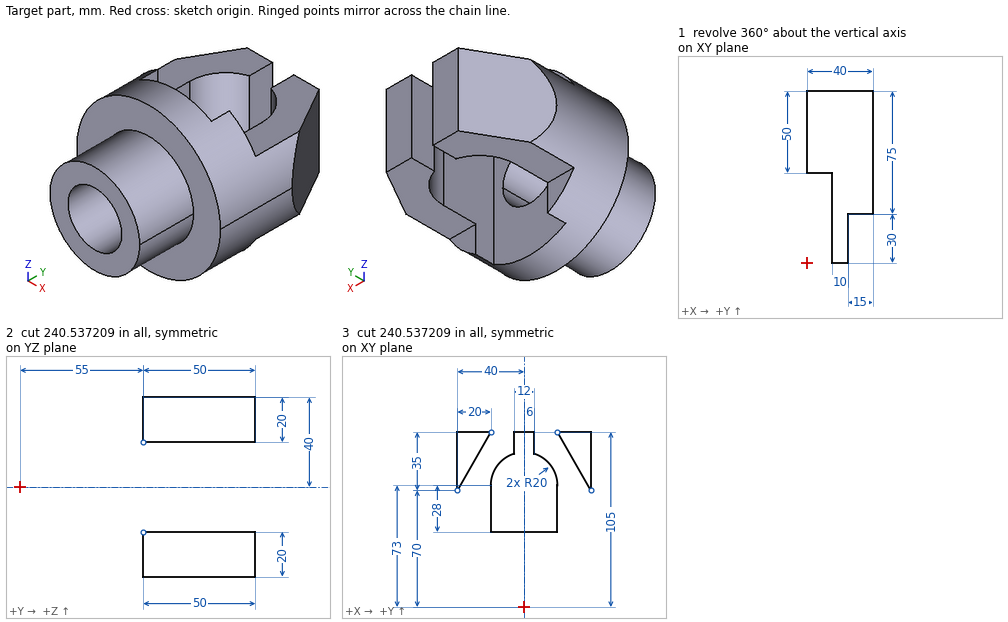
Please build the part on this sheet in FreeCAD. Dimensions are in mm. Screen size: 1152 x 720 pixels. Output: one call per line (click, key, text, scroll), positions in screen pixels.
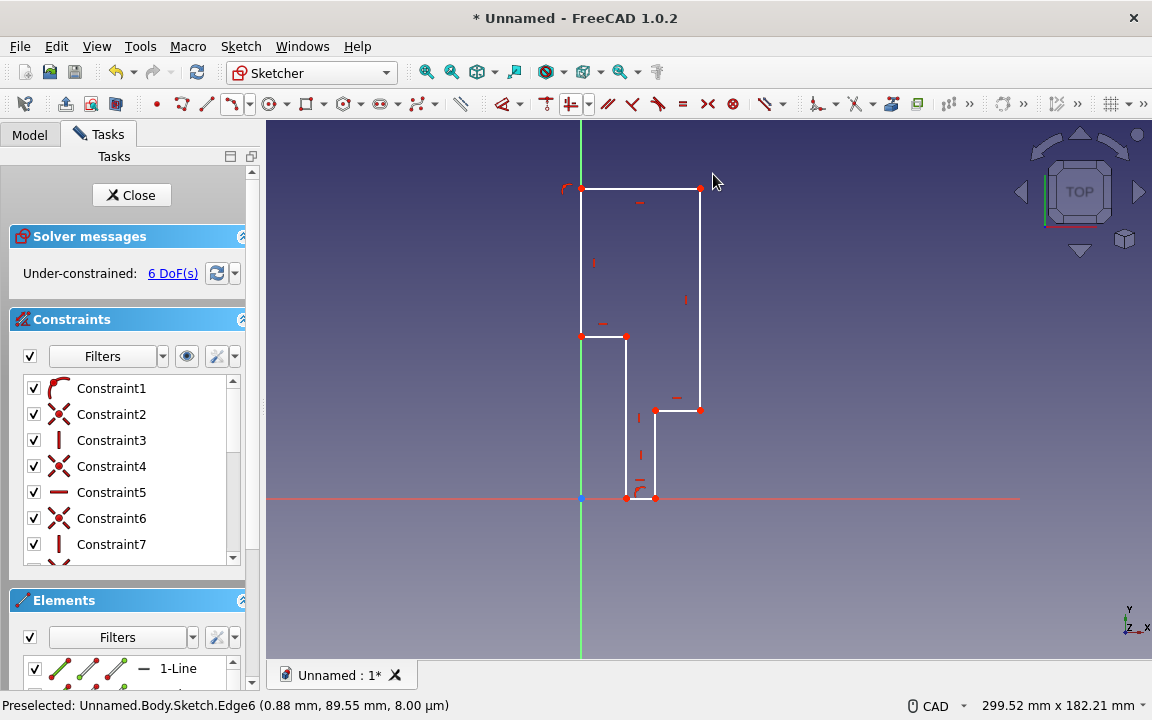
click(502, 104)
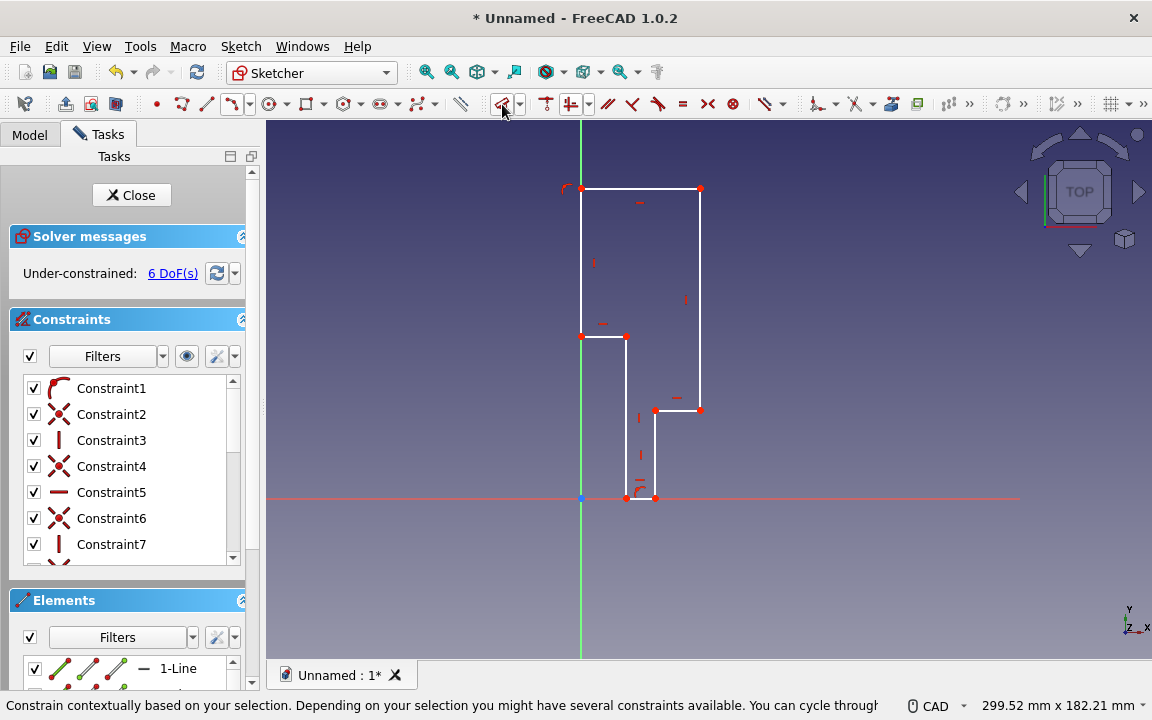
scroll(638, 499, up, 2)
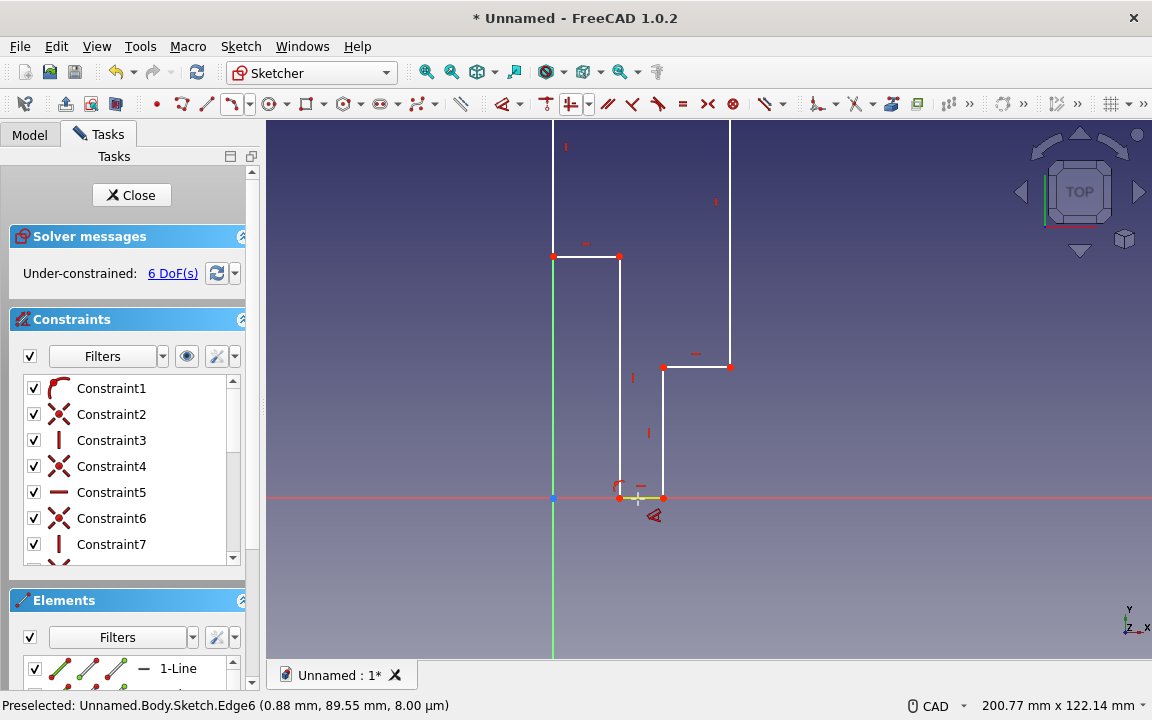
click(637, 498)
click(642, 532)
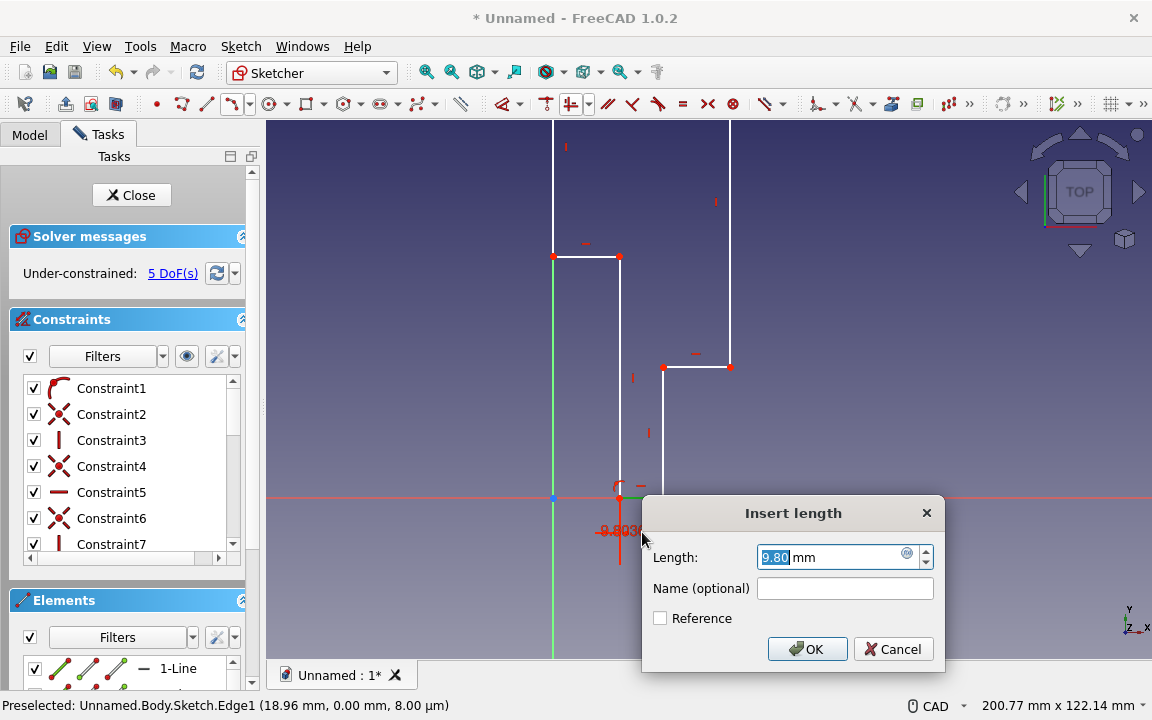
text(10)
key(Return)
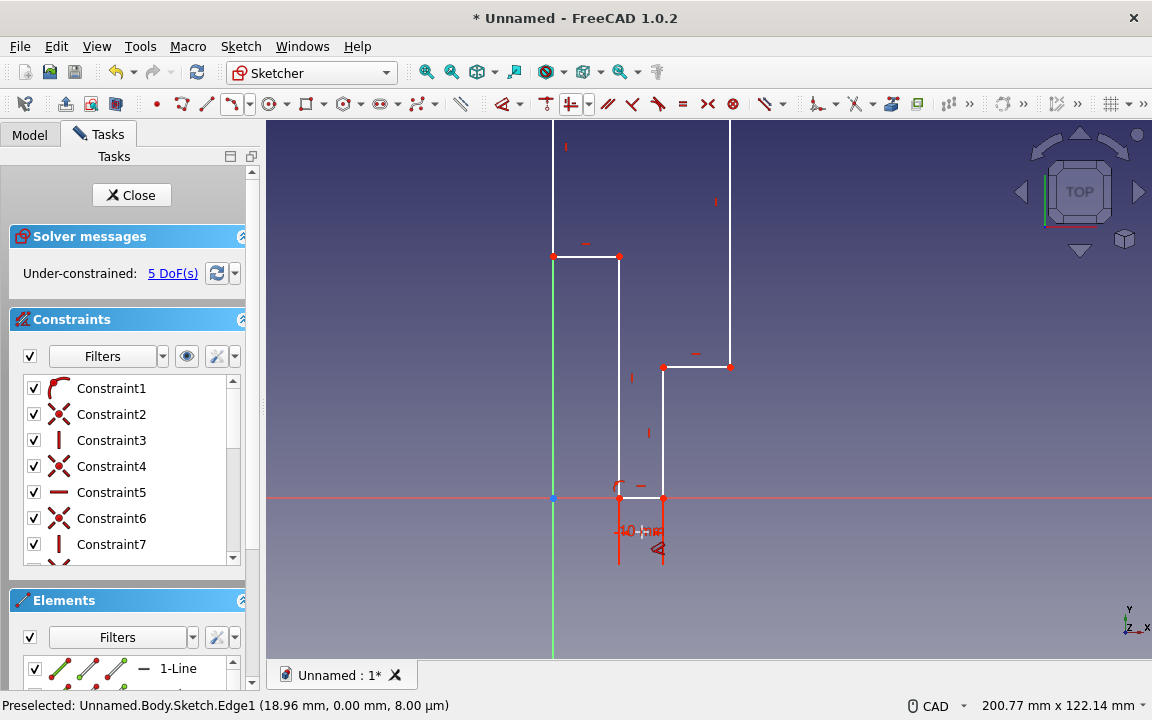
click(663, 459)
click(697, 433)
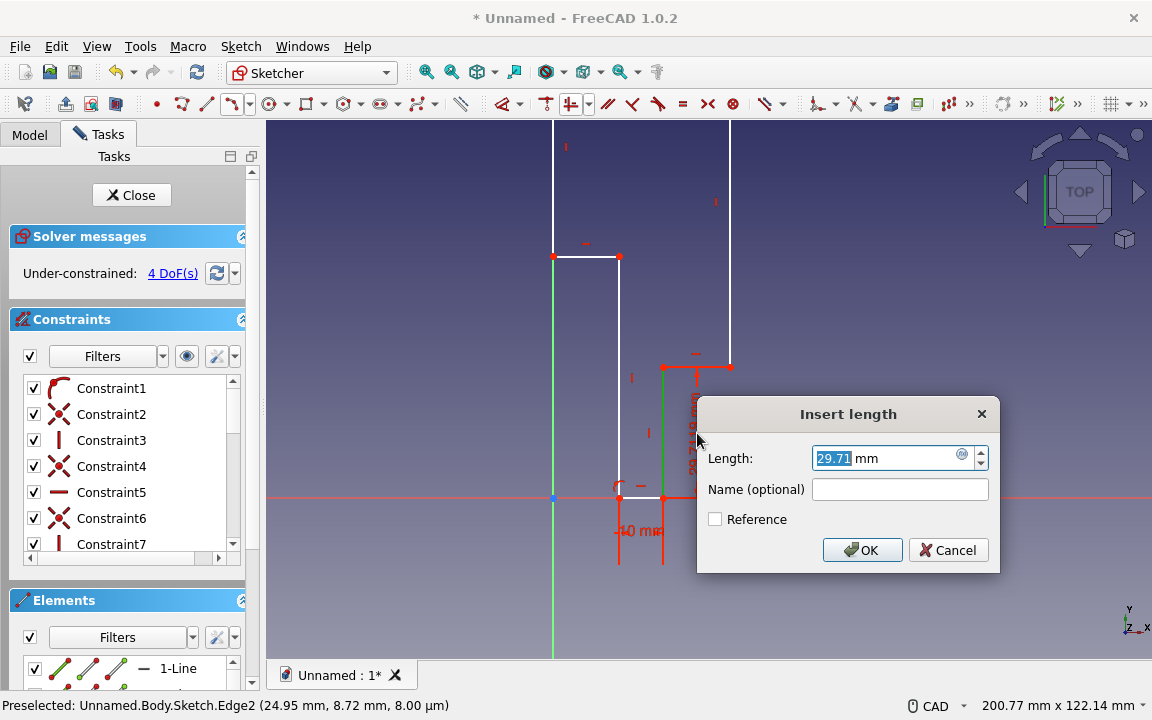
text(30)
key(Return)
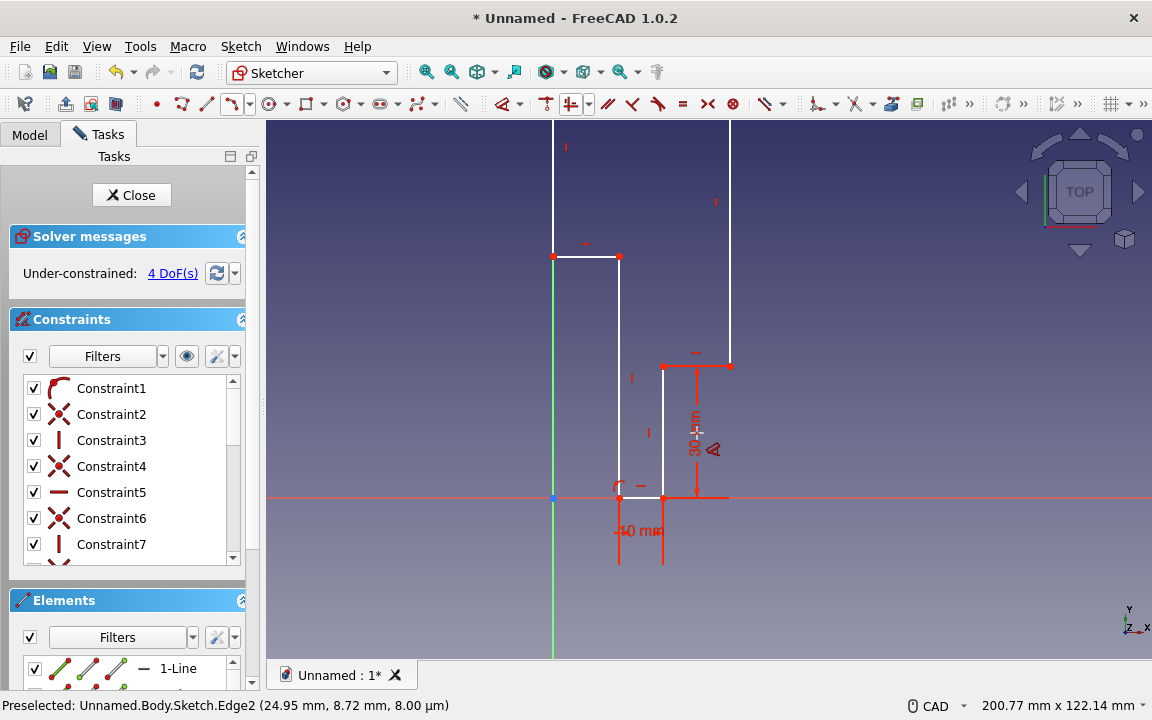
click(684, 366)
click(697, 400)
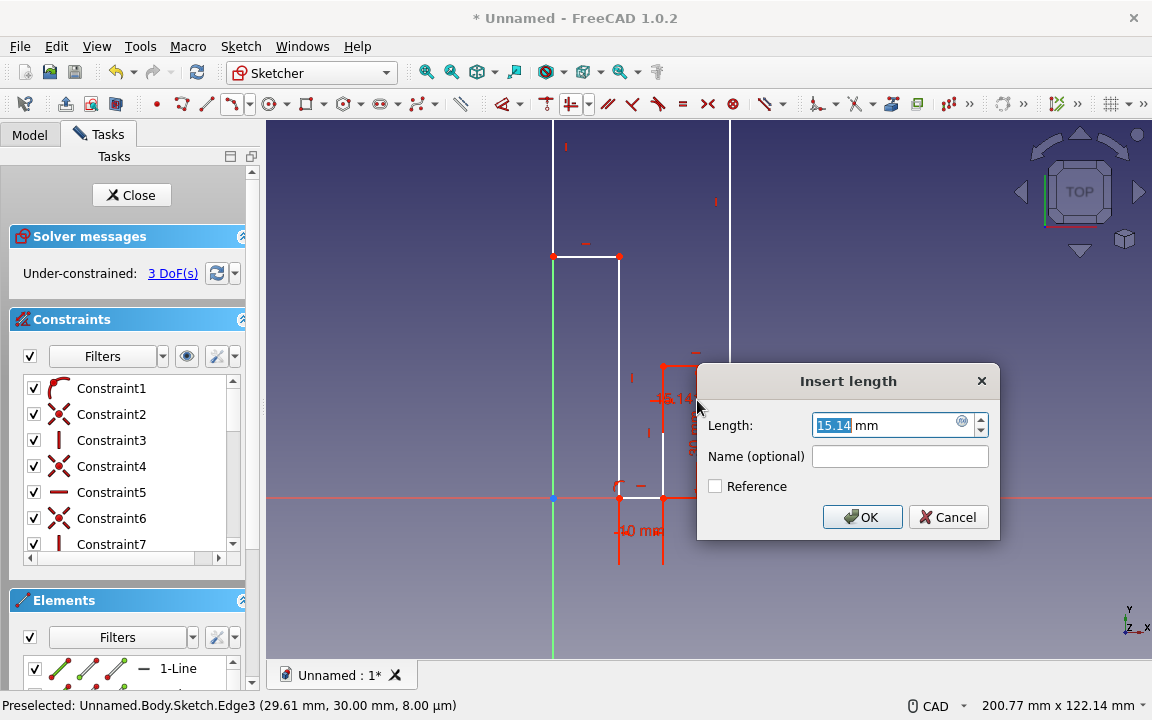
text(15)
key(Return)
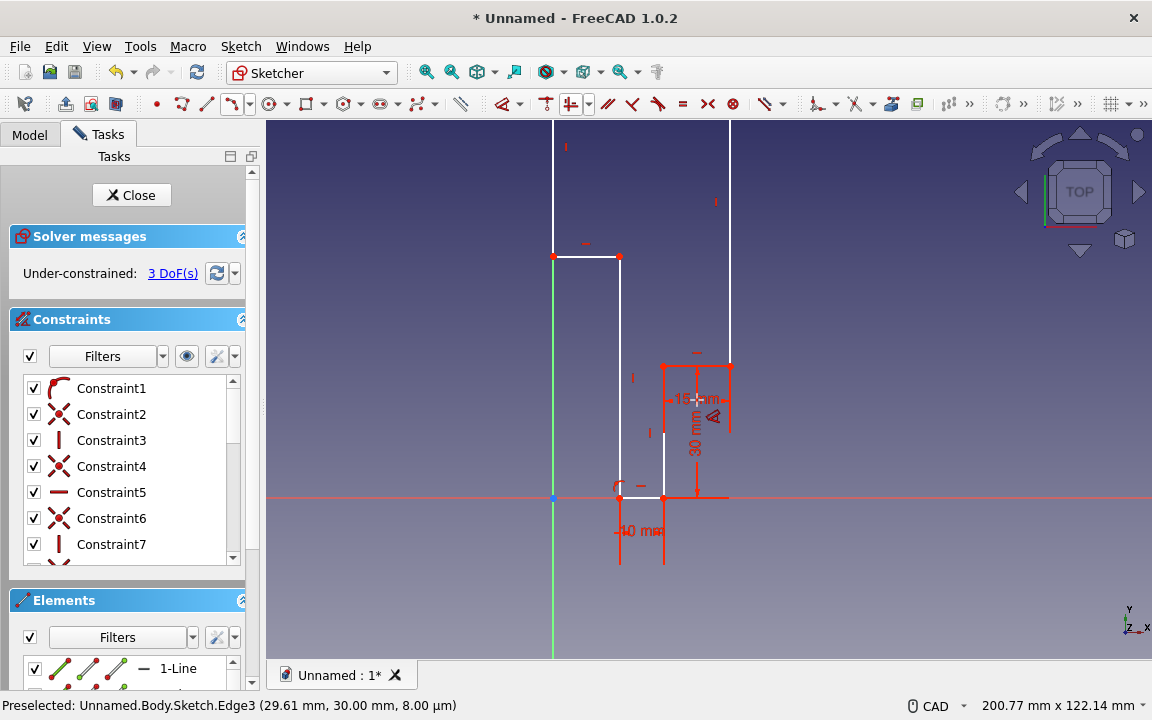
click(730, 267)
click(764, 257)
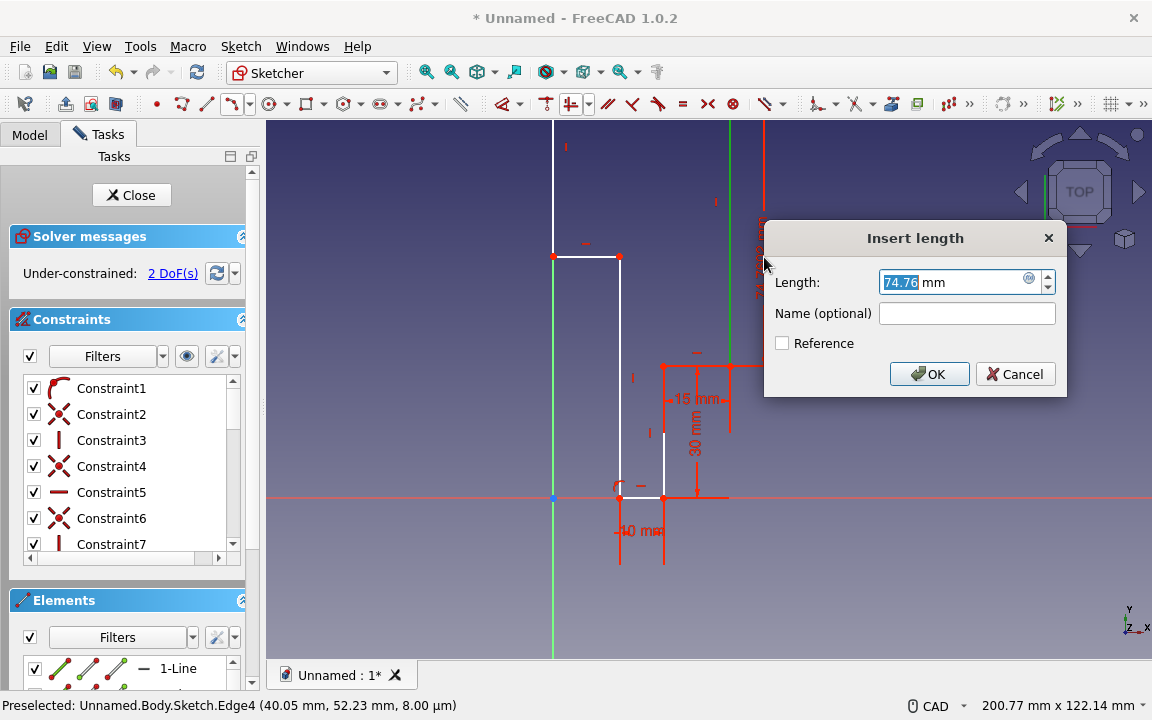
text(75)
key(Return)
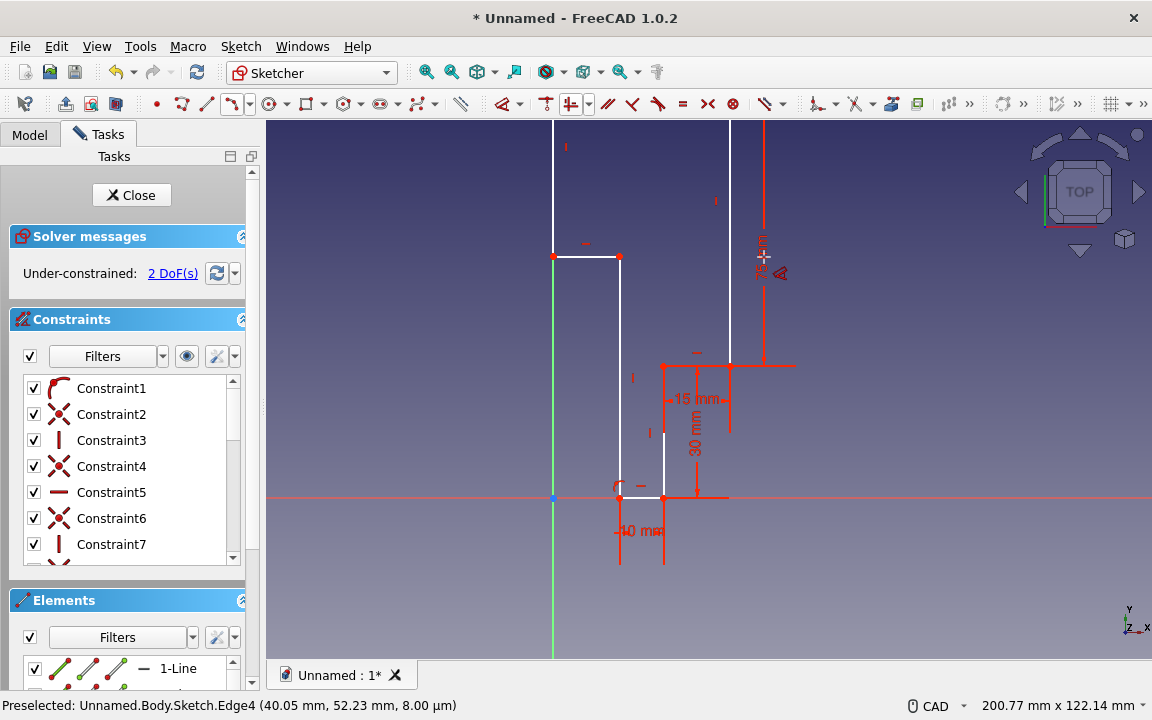
scroll(638, 631, down, 2)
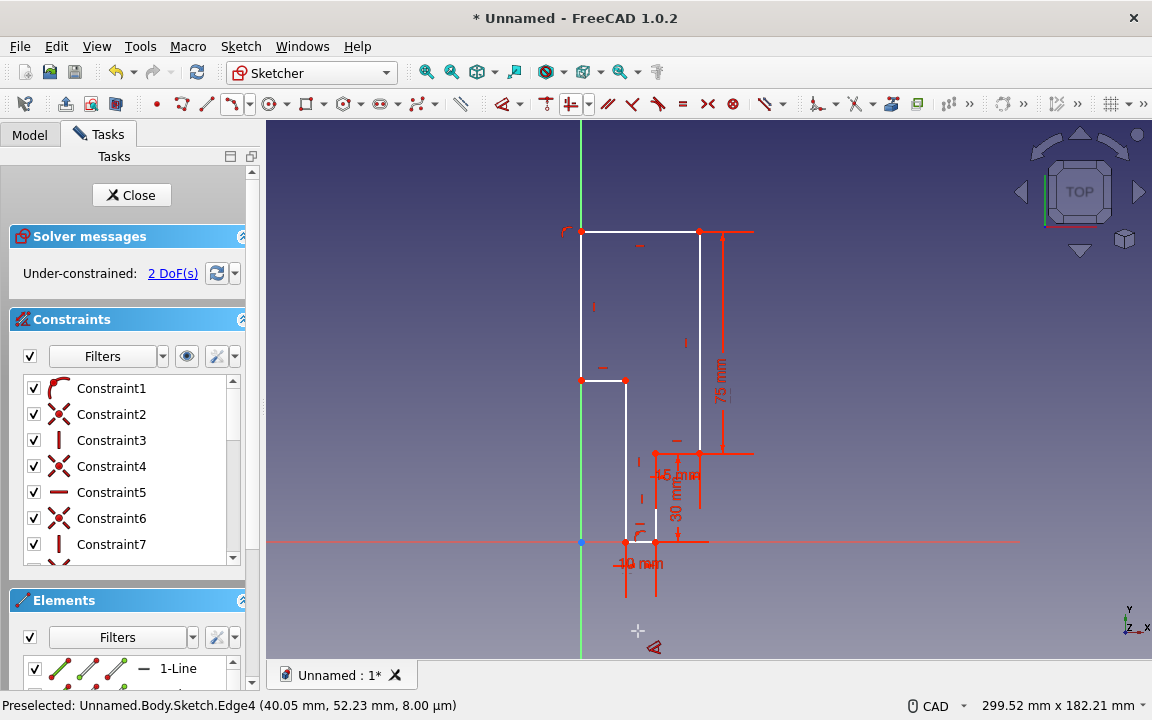
click(664, 232)
click(641, 198)